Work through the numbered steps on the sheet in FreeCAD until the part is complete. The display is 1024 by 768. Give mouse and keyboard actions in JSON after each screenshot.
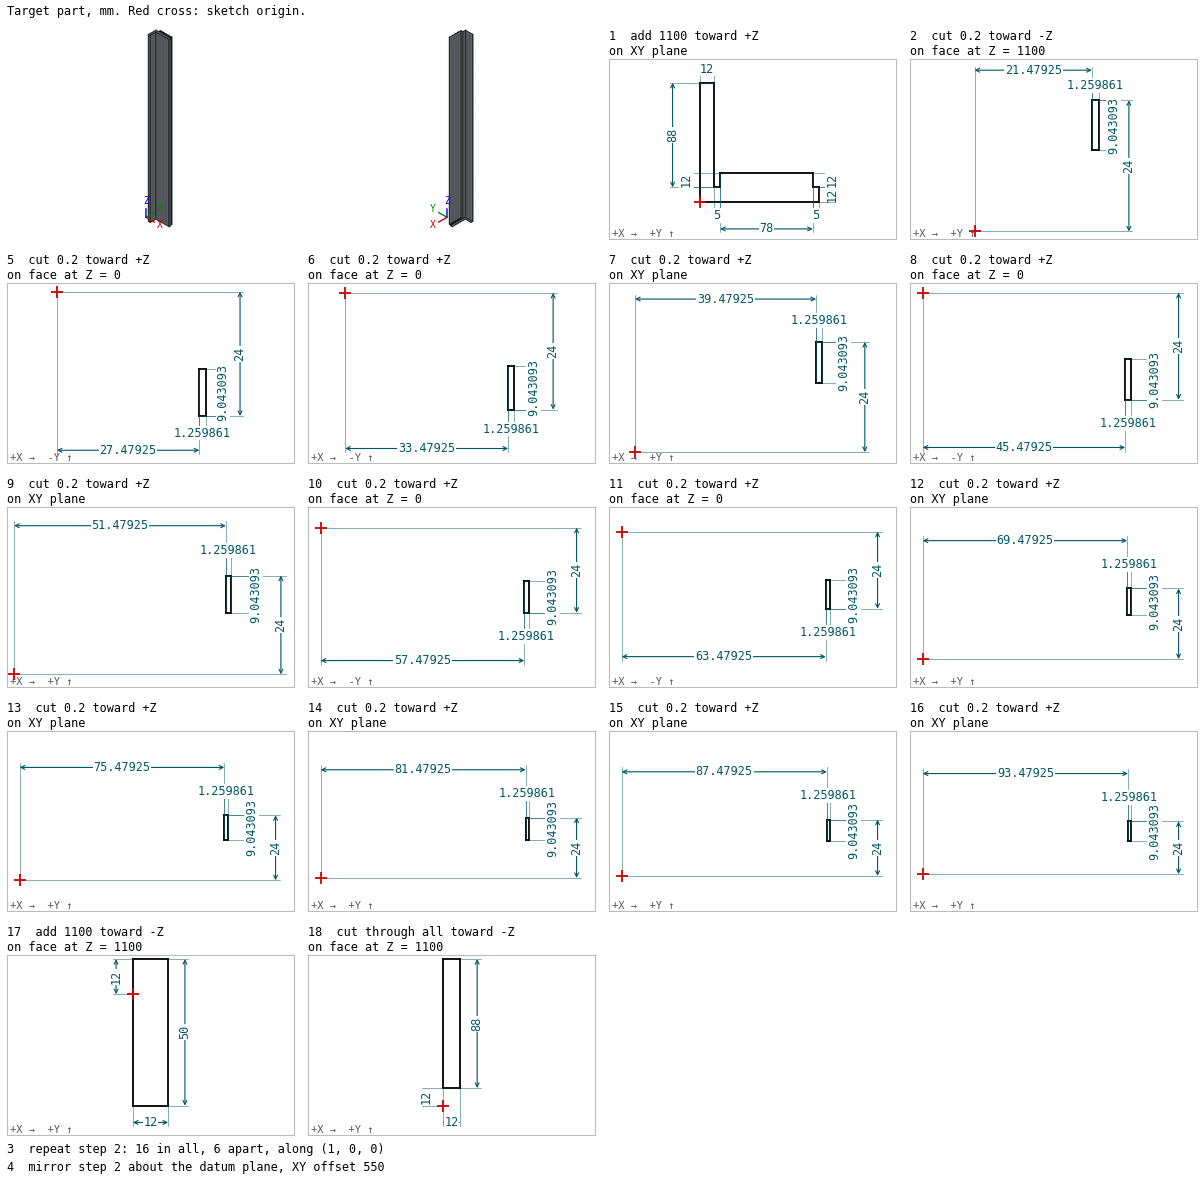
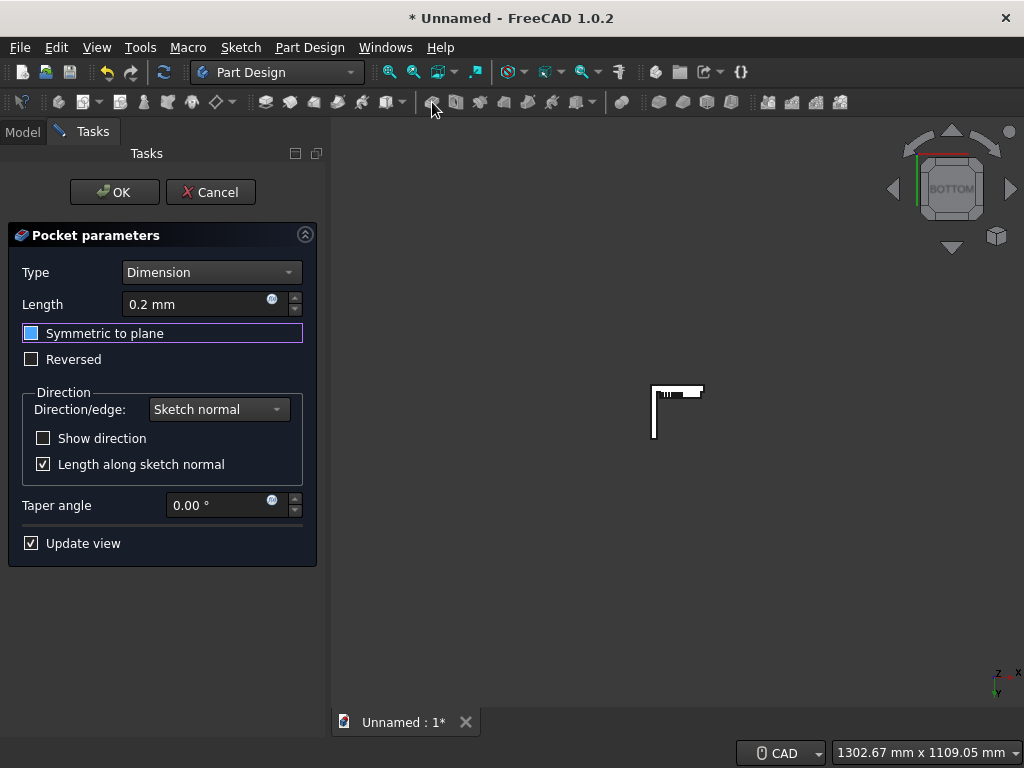
{"action": "left_click", "coordinate": [115, 192]}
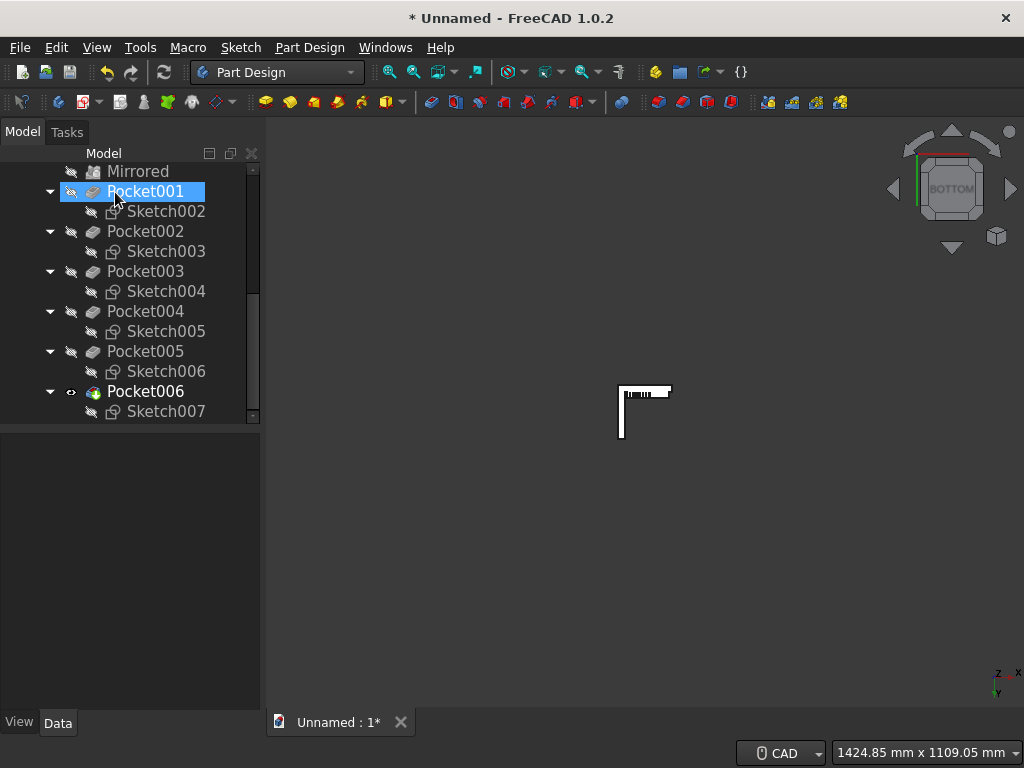
{"action": "left_click", "coordinate": [390, 72]}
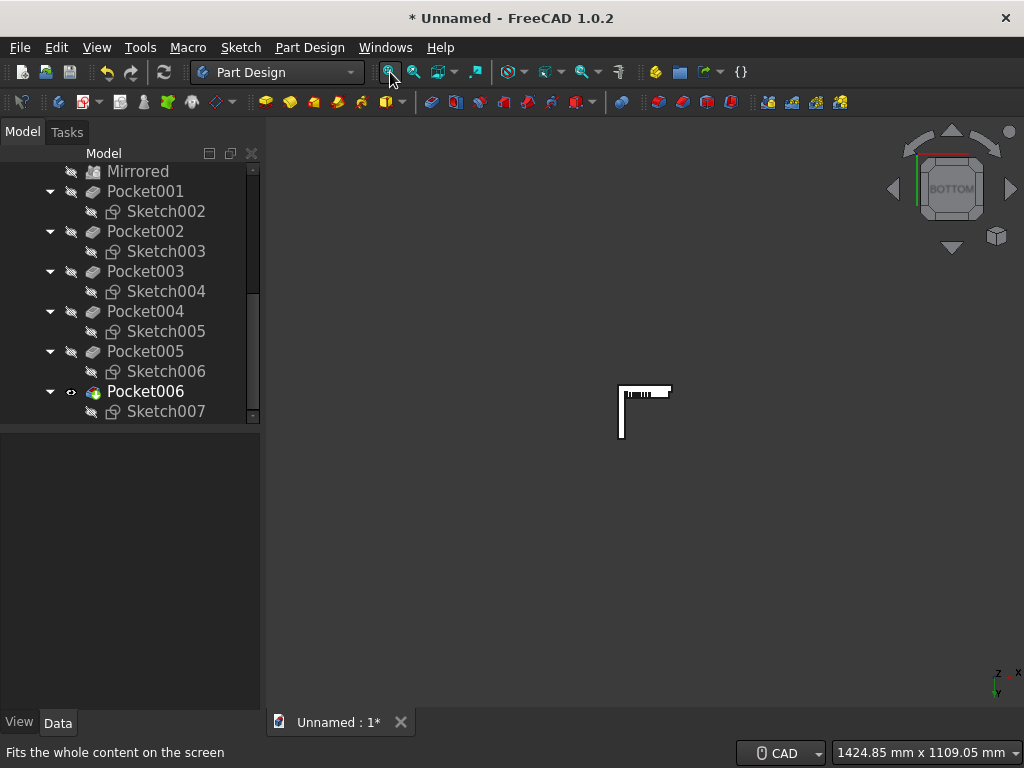
{"action": "left_click", "coordinate": [660, 388]}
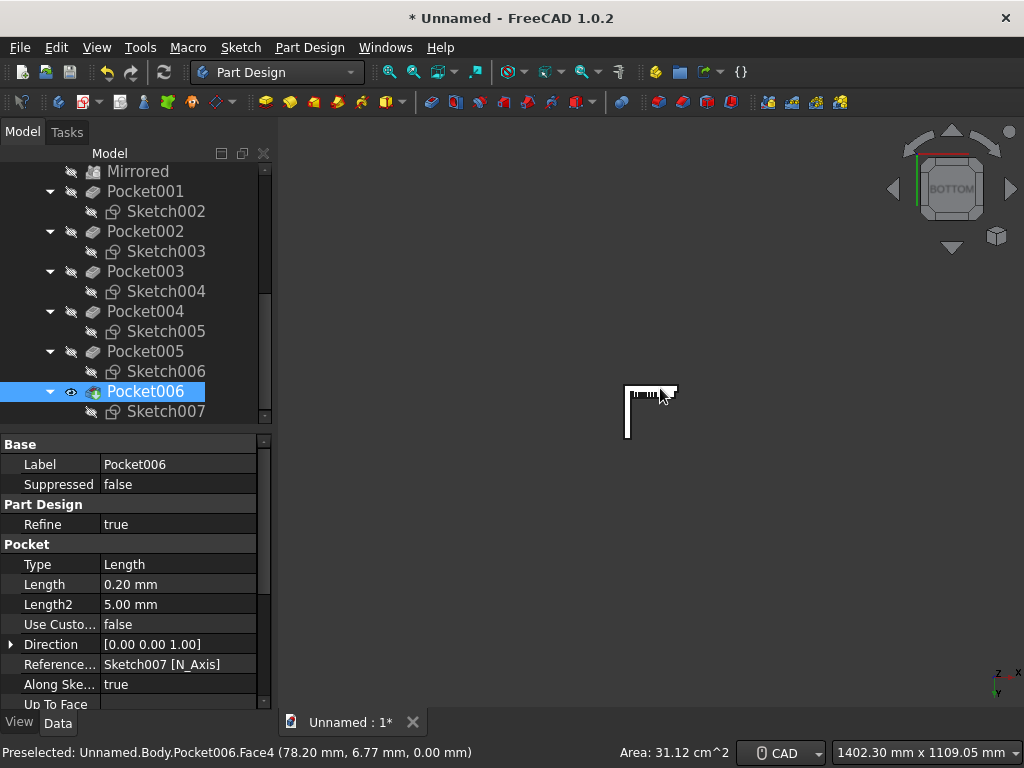
{"action": "left_click", "coordinate": [84, 102]}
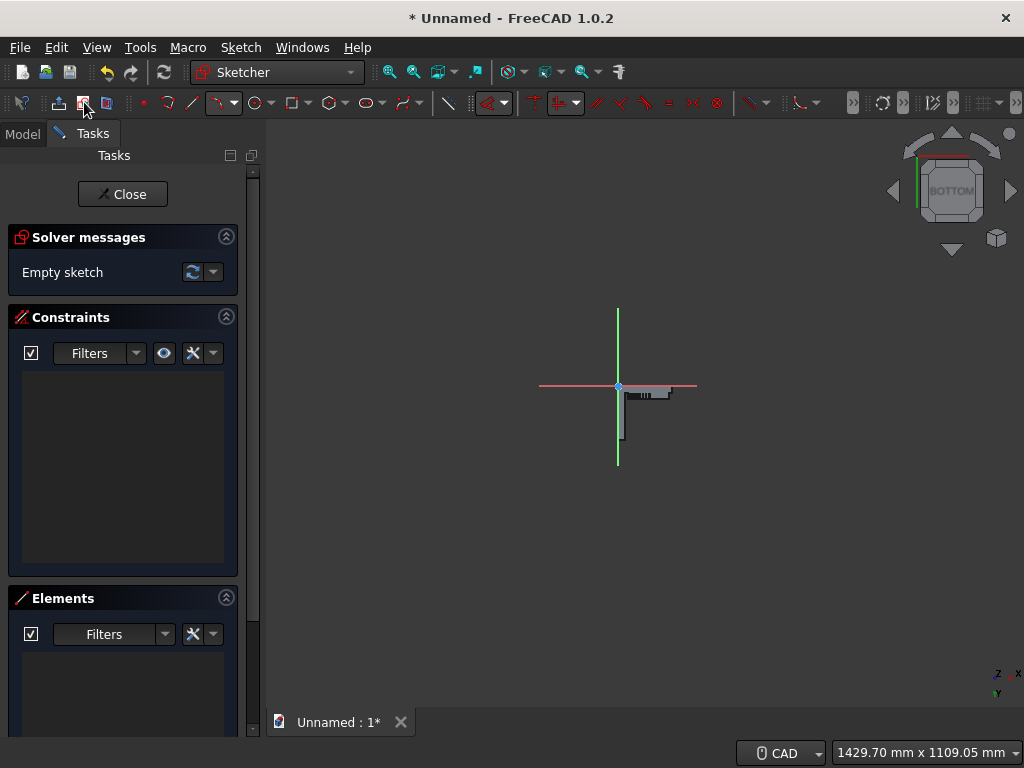
{"action": "scroll", "coordinate": [656, 396], "scroll_direction": "up", "scroll_amount": 15}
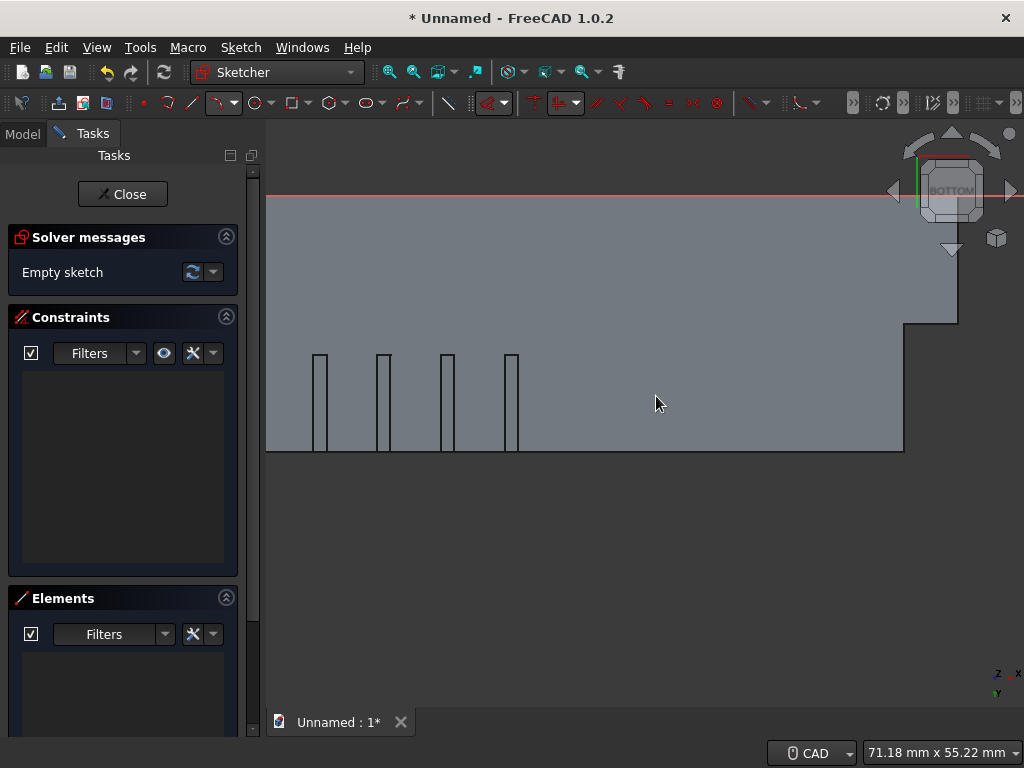
{"action": "scroll", "coordinate": [575, 400], "scroll_direction": "up", "scroll_amount": 7}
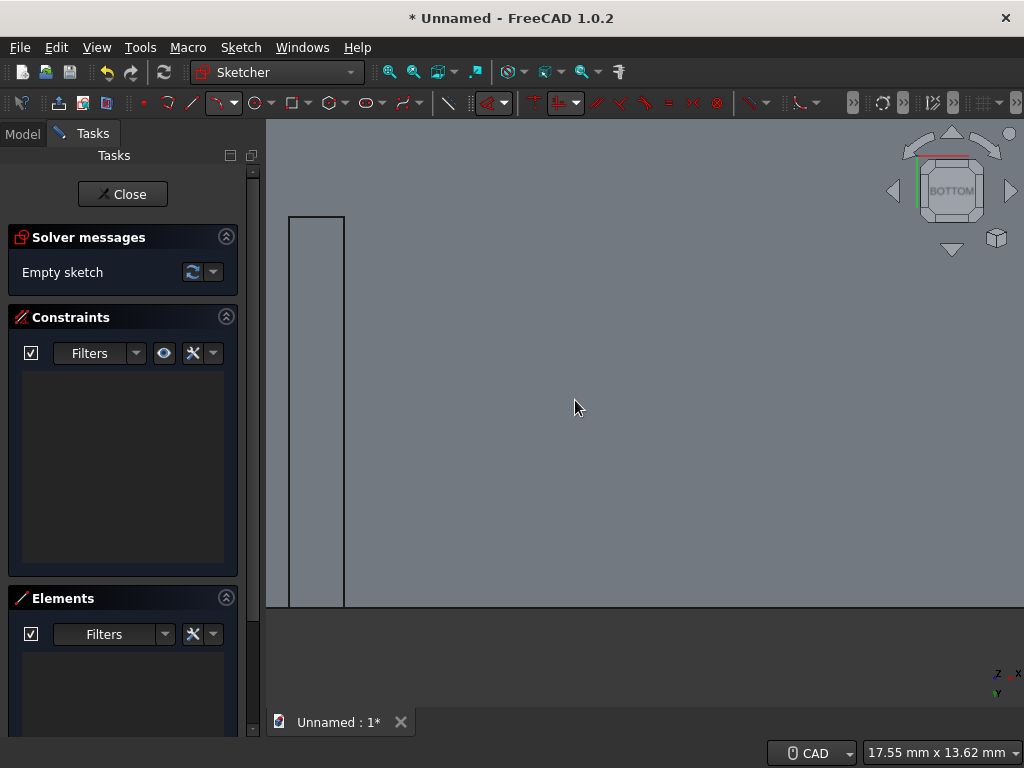
{"action": "left_click", "coordinate": [292, 104]}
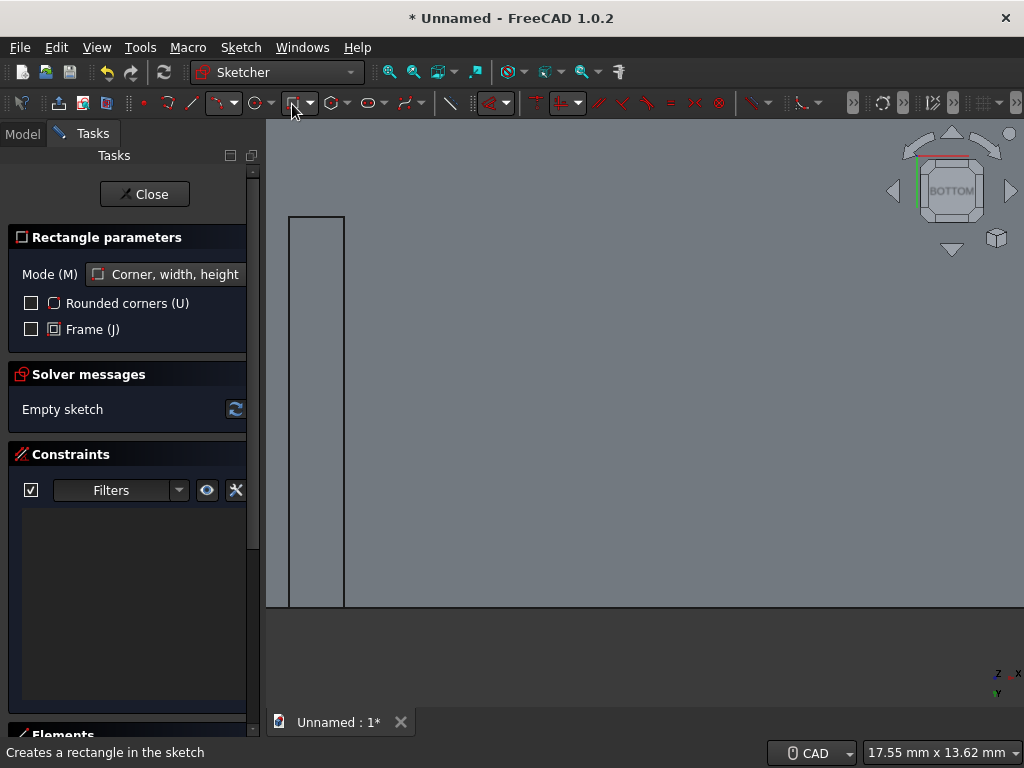
{"action": "left_click", "coordinate": [548, 217]}
{"action": "mouse_move", "coordinate": [603, 608]}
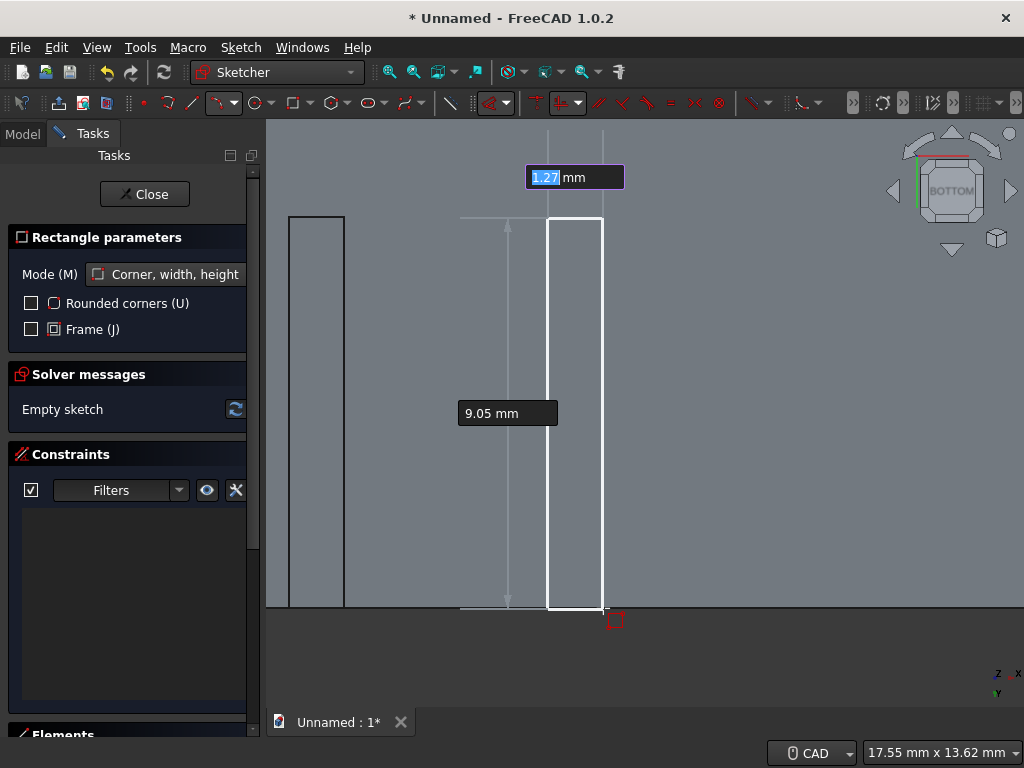
{"action": "type", "text": "1.259861"}
{"action": "key", "text": "Tab"}
{"action": "type", "text": "9.043093"}
{"action": "key", "text": "Return"}
{"action": "key", "text": "Escape"}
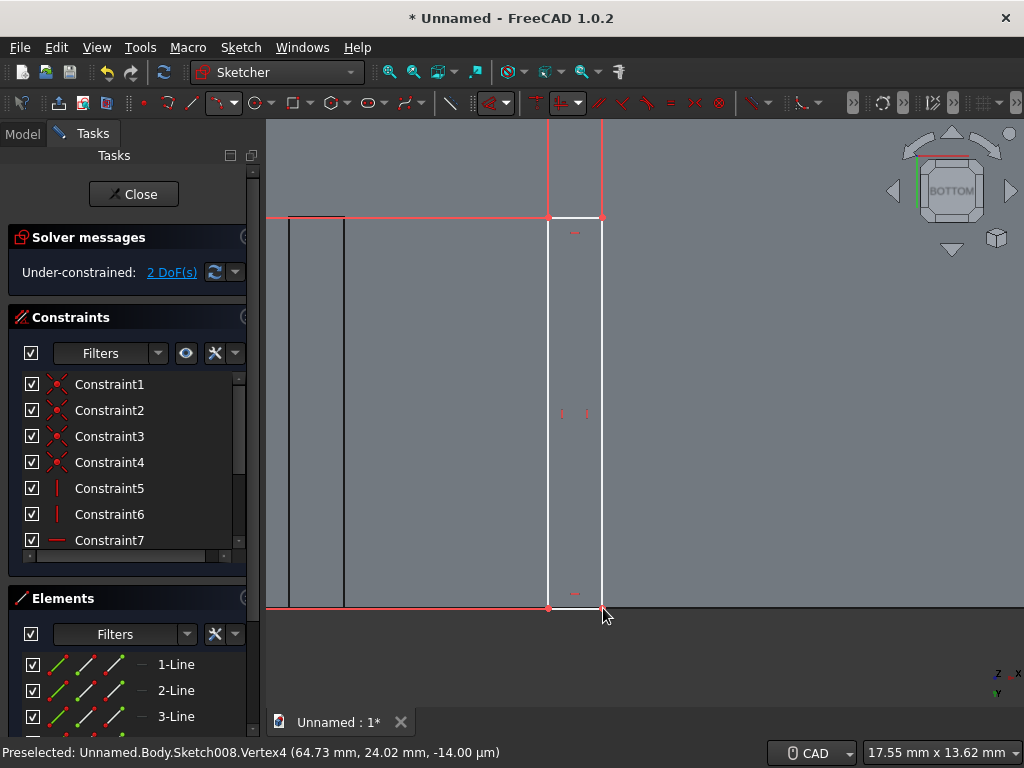
{"action": "left_click", "coordinate": [548, 609]}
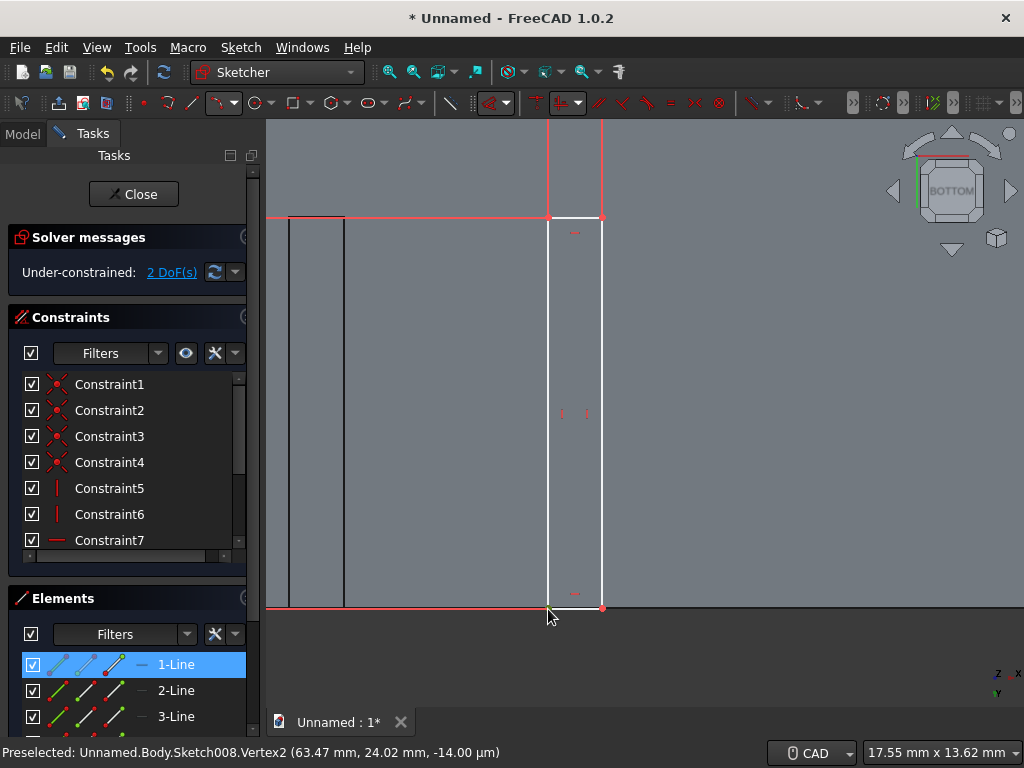
{"action": "left_click", "coordinate": [508, 104]}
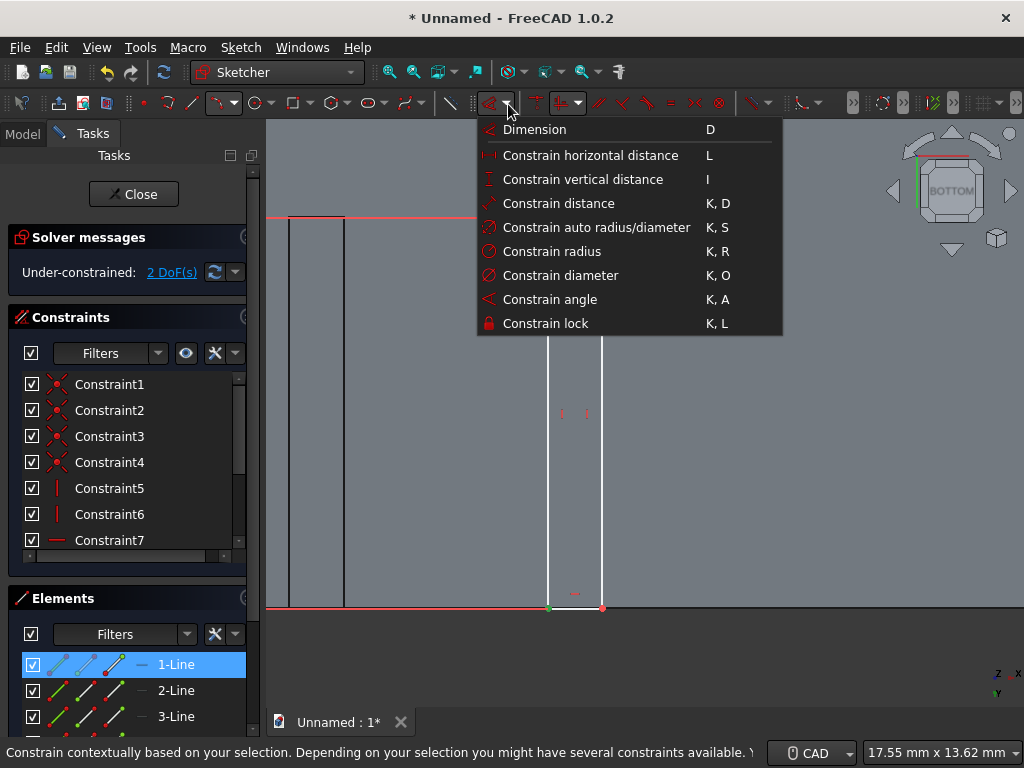
{"action": "left_click", "coordinate": [630, 179]}